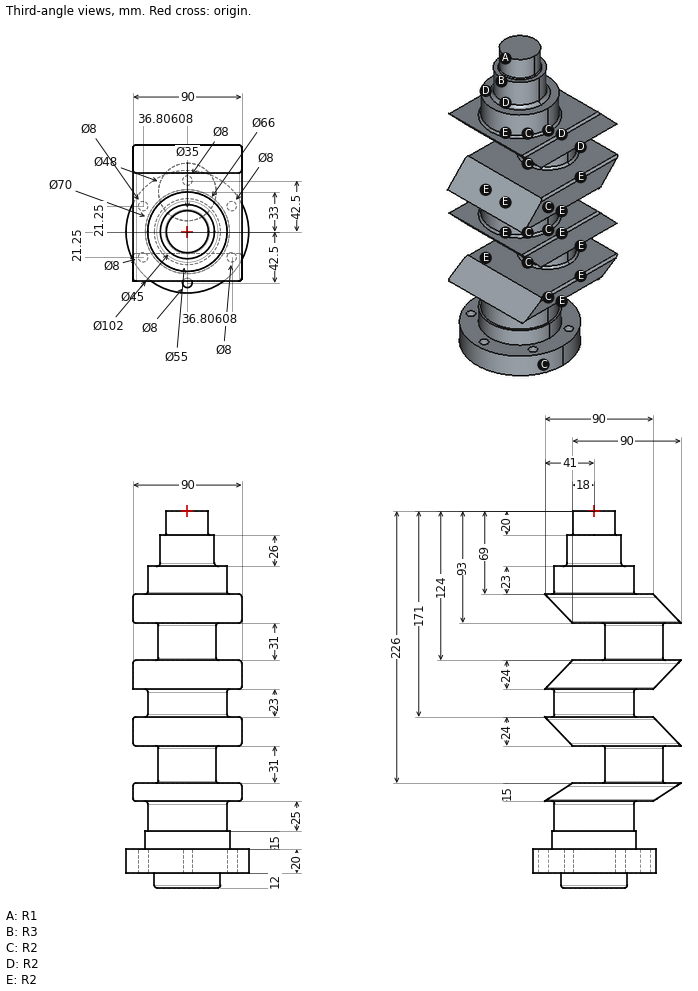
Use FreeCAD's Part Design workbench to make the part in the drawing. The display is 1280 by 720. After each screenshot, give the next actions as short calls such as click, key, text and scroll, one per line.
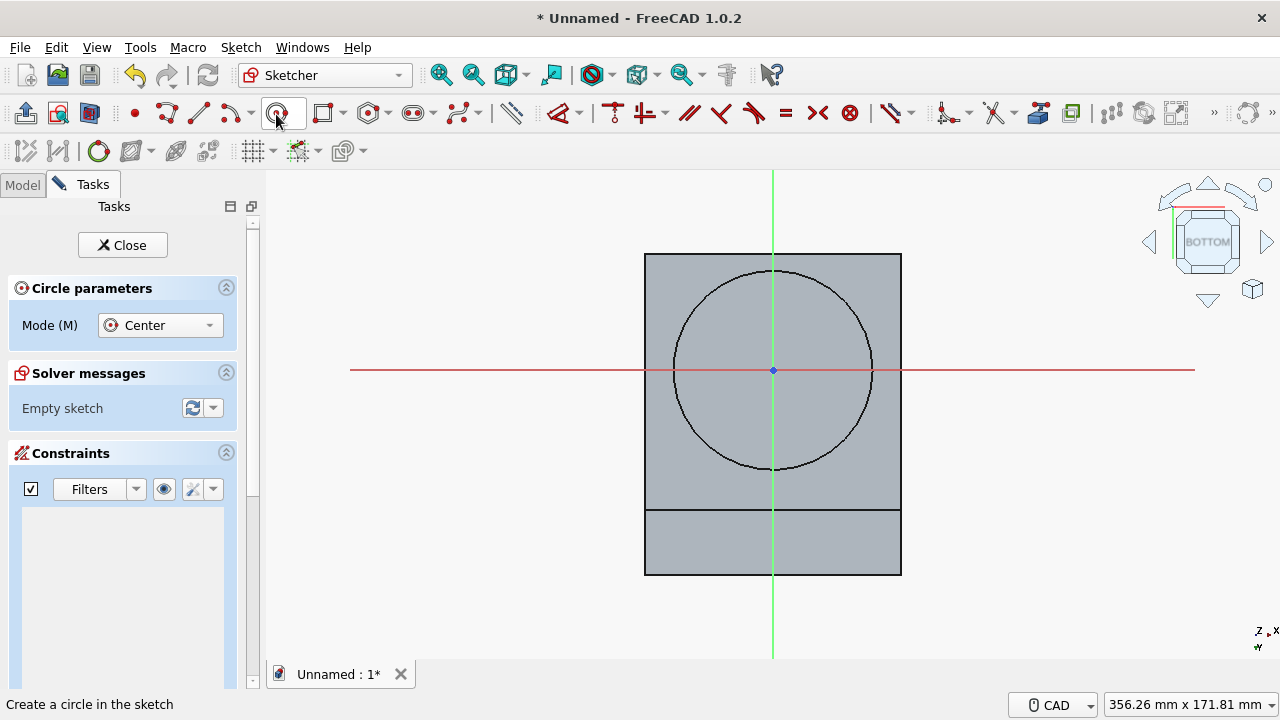
click(773, 370)
move(876, 268)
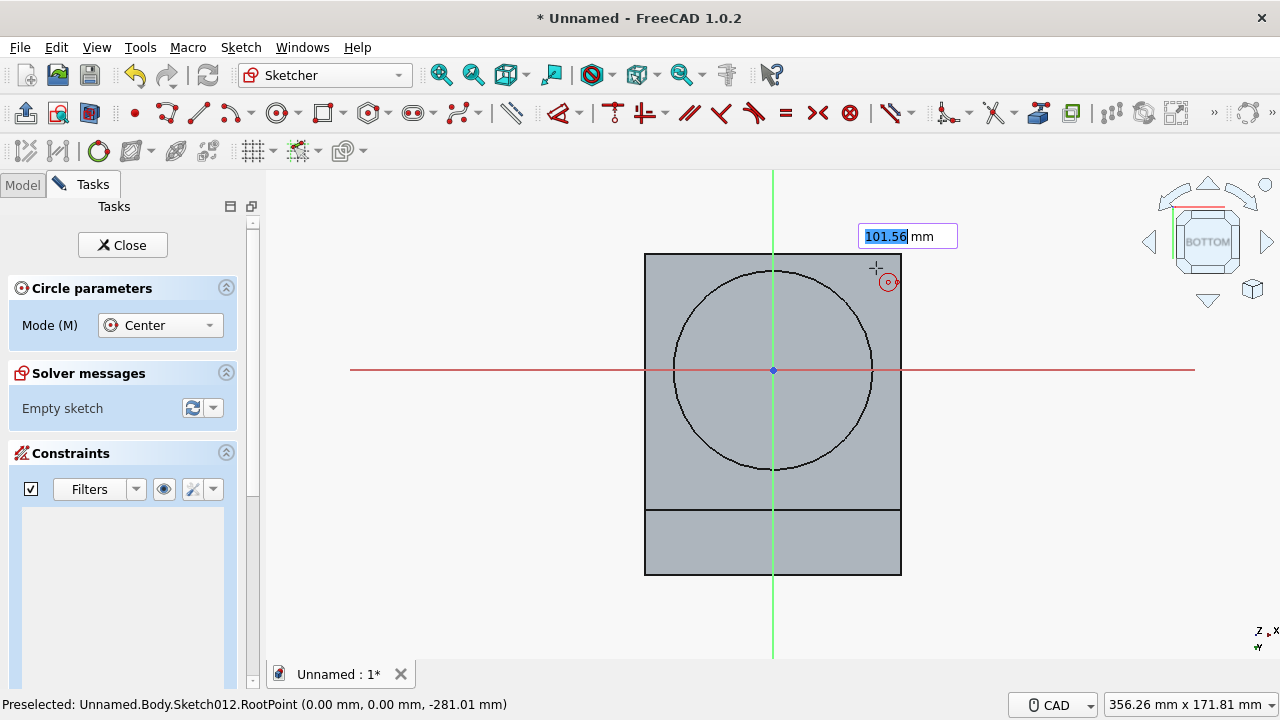
text(102)
key(Return)
key(Escape)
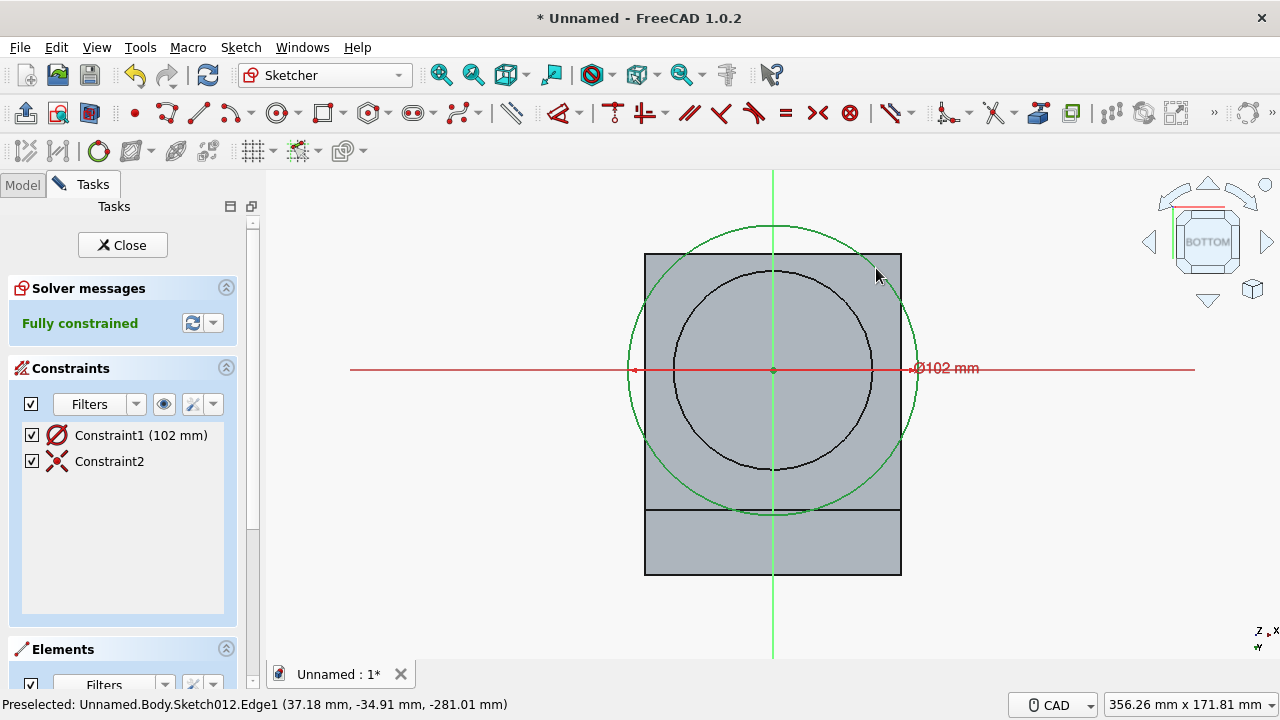
click(123, 245)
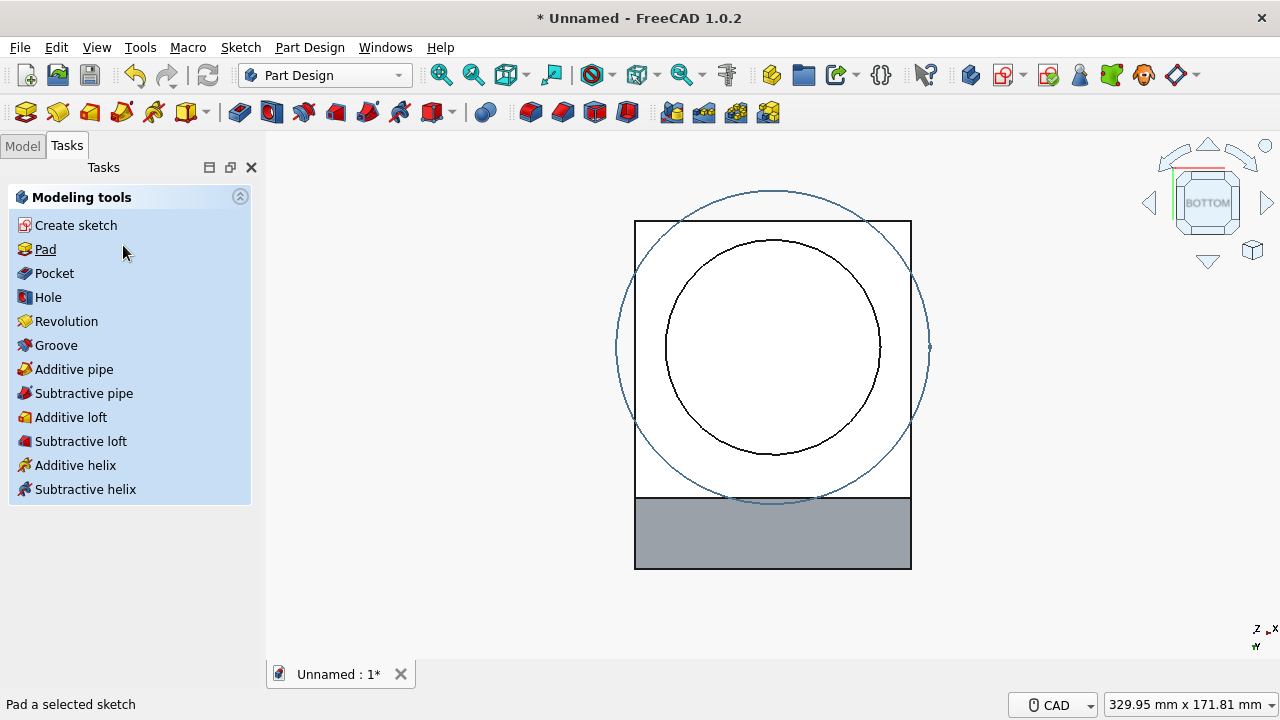
click(26, 112)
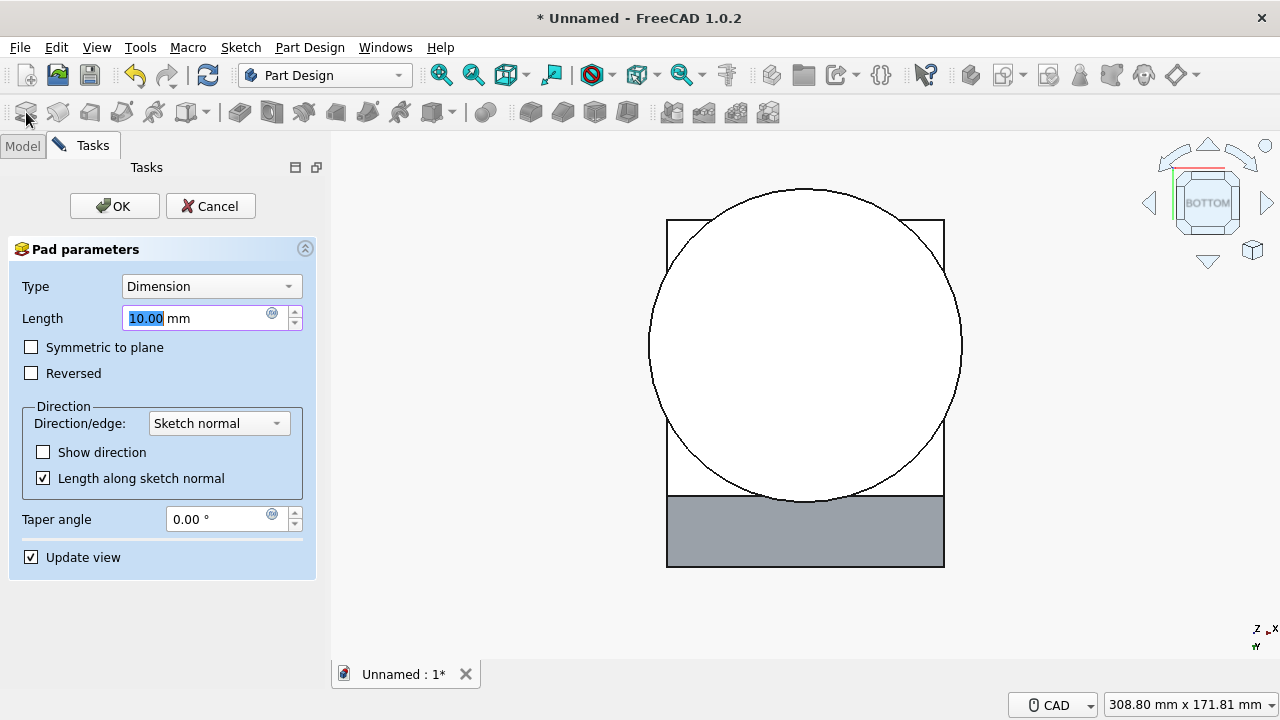
text(20)
key(Tab)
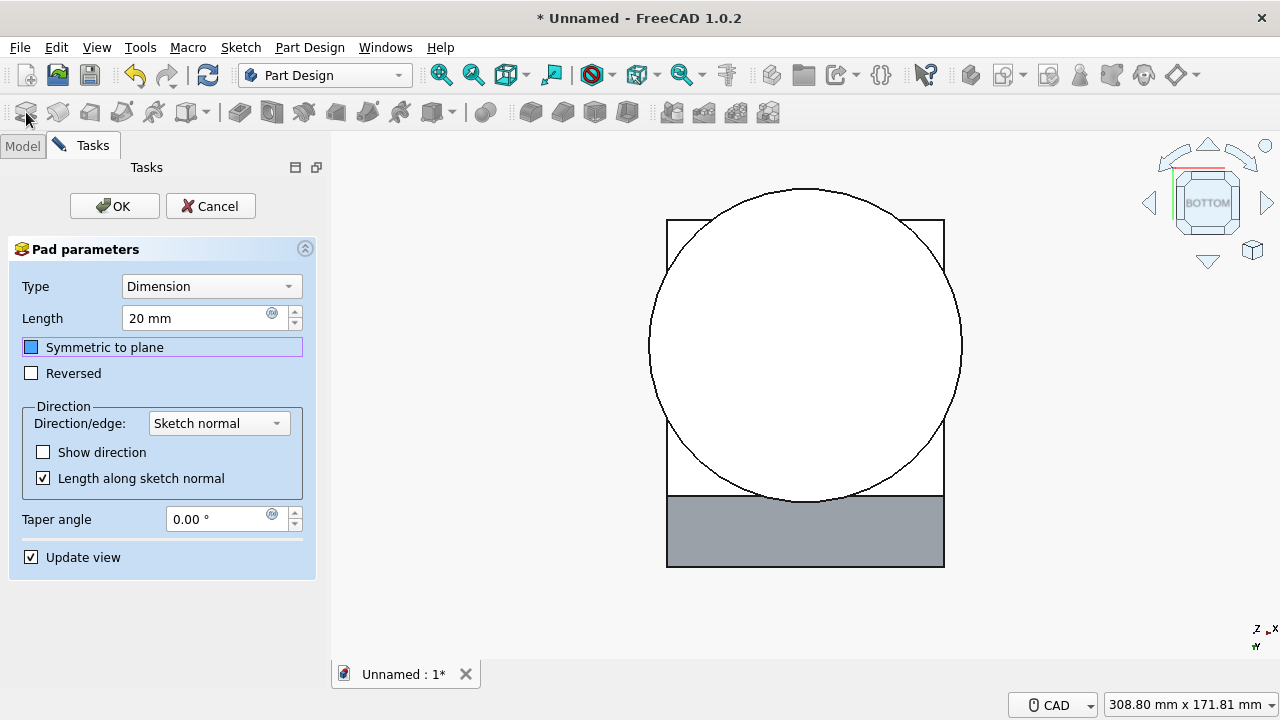
click(115, 206)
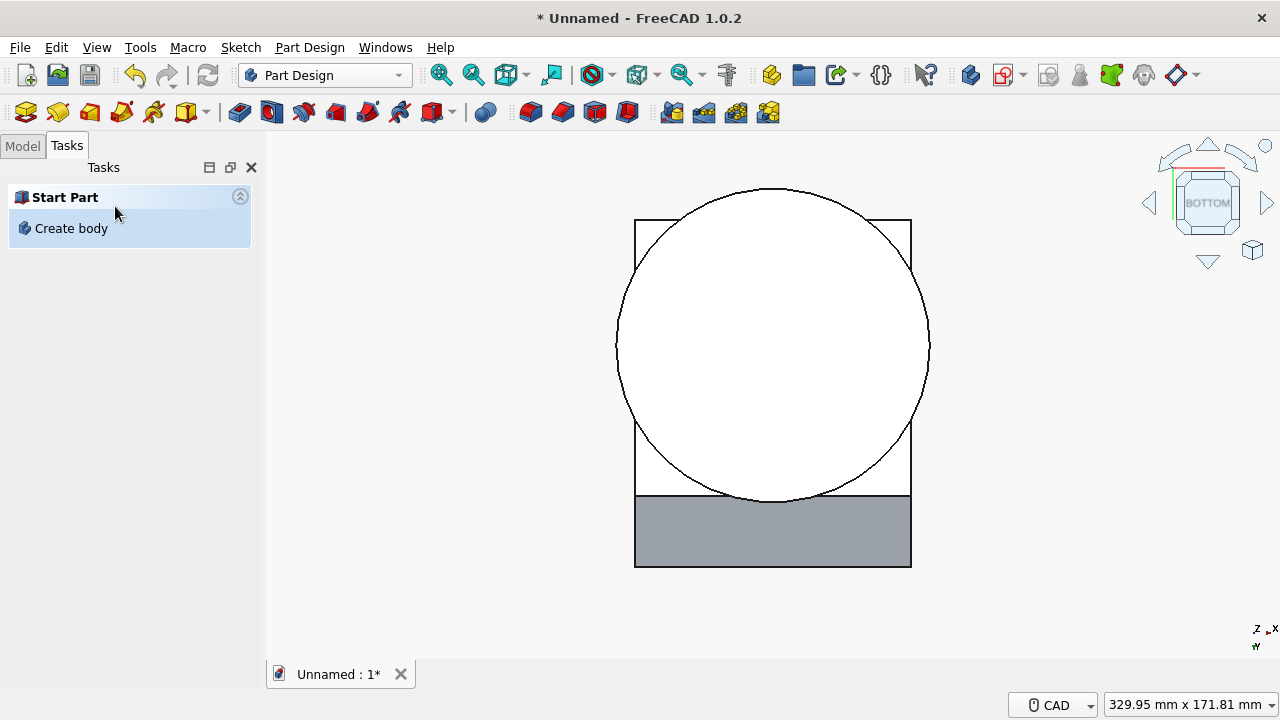
click(773, 345)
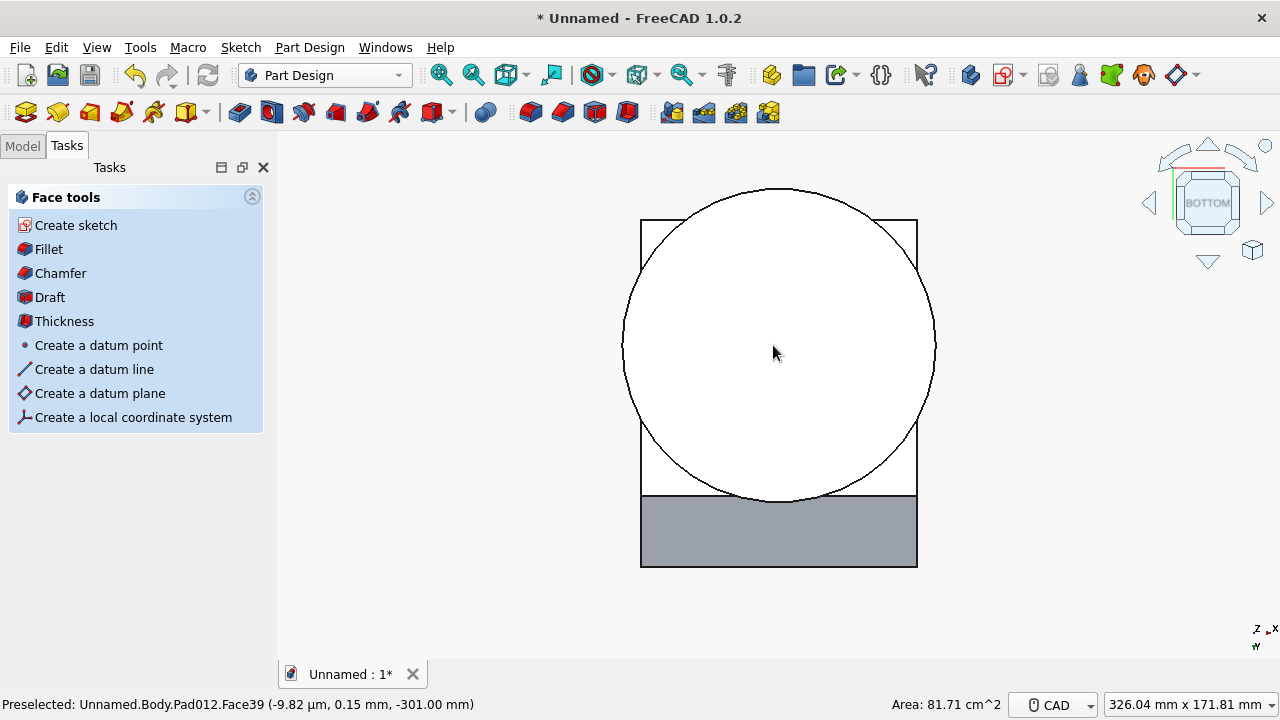
click(1004, 76)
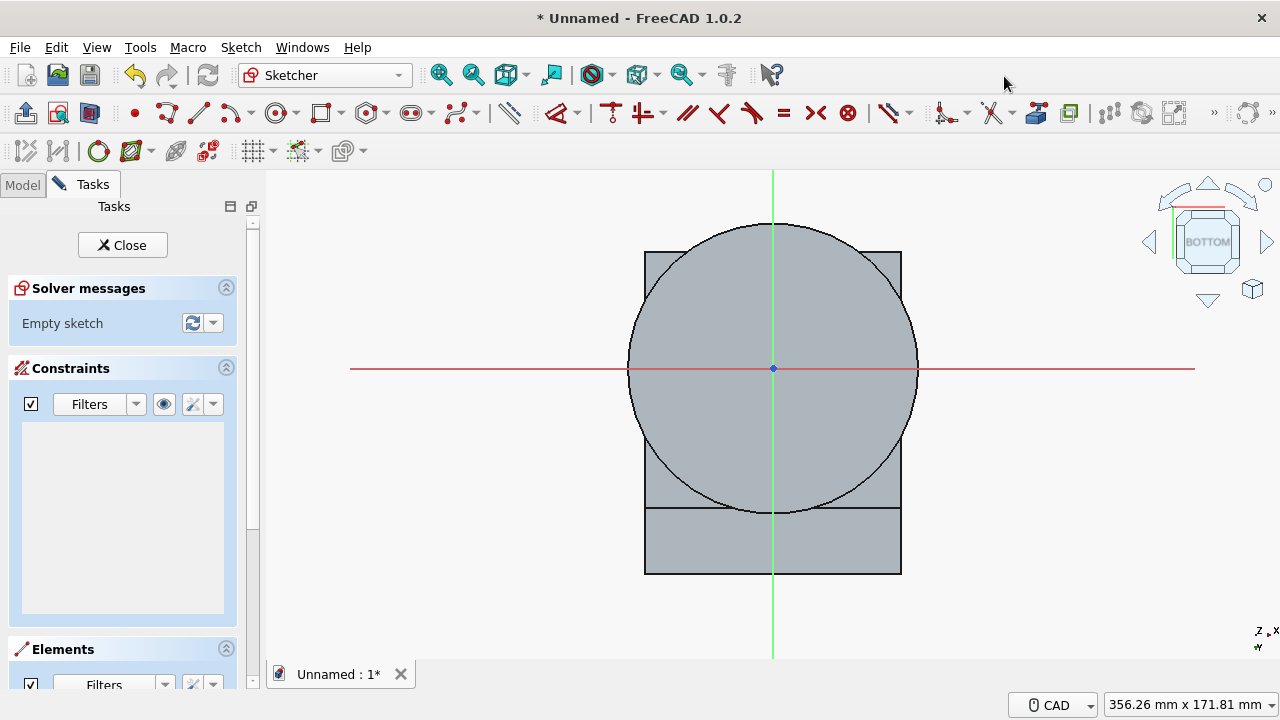
scroll(856, 313, up, 3)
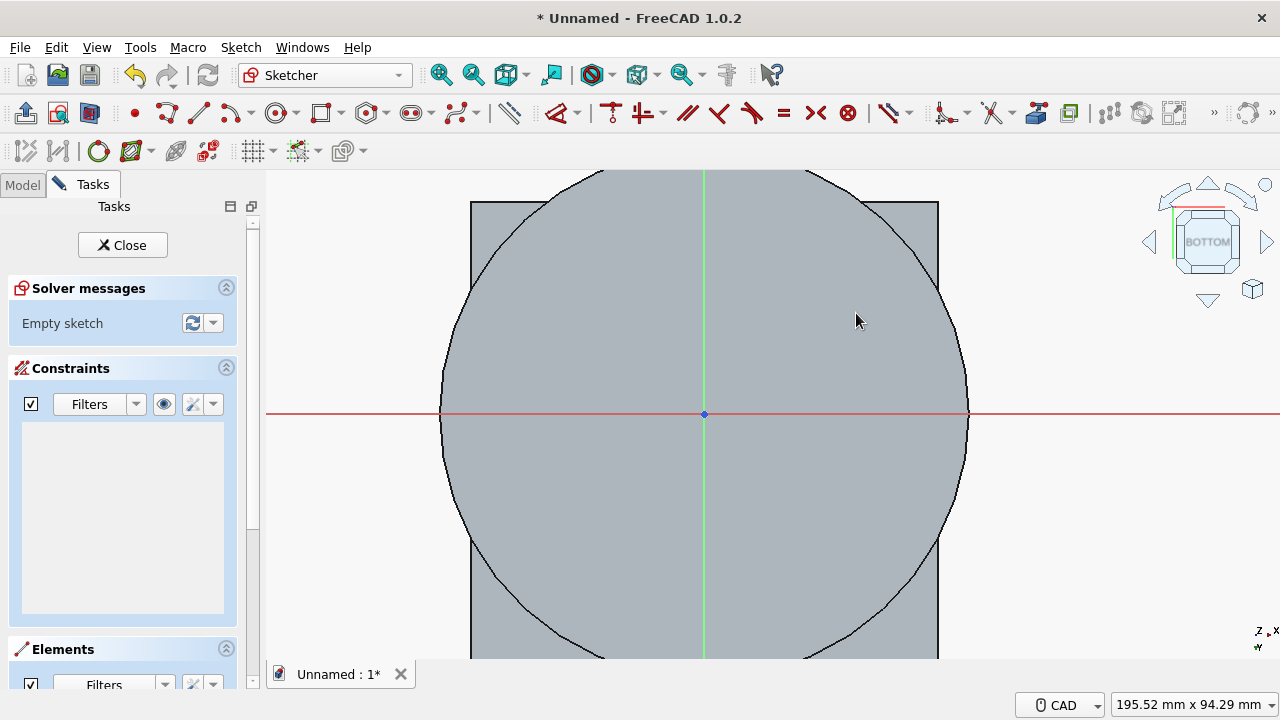
click(276, 114)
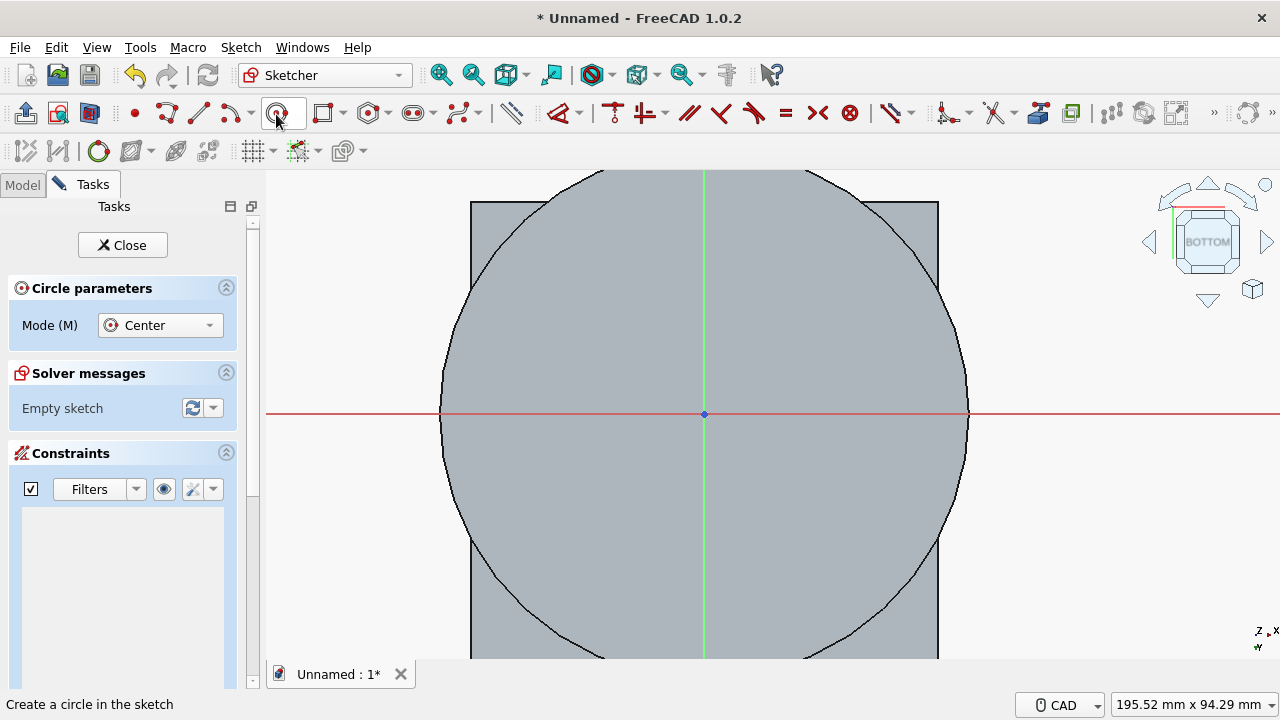
click(704, 414)
move(805, 313)